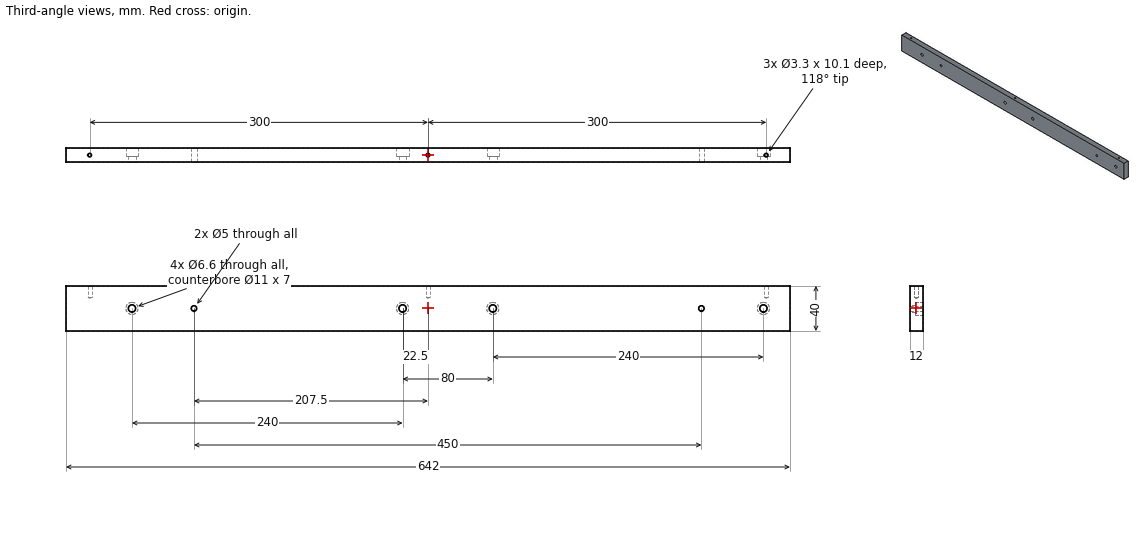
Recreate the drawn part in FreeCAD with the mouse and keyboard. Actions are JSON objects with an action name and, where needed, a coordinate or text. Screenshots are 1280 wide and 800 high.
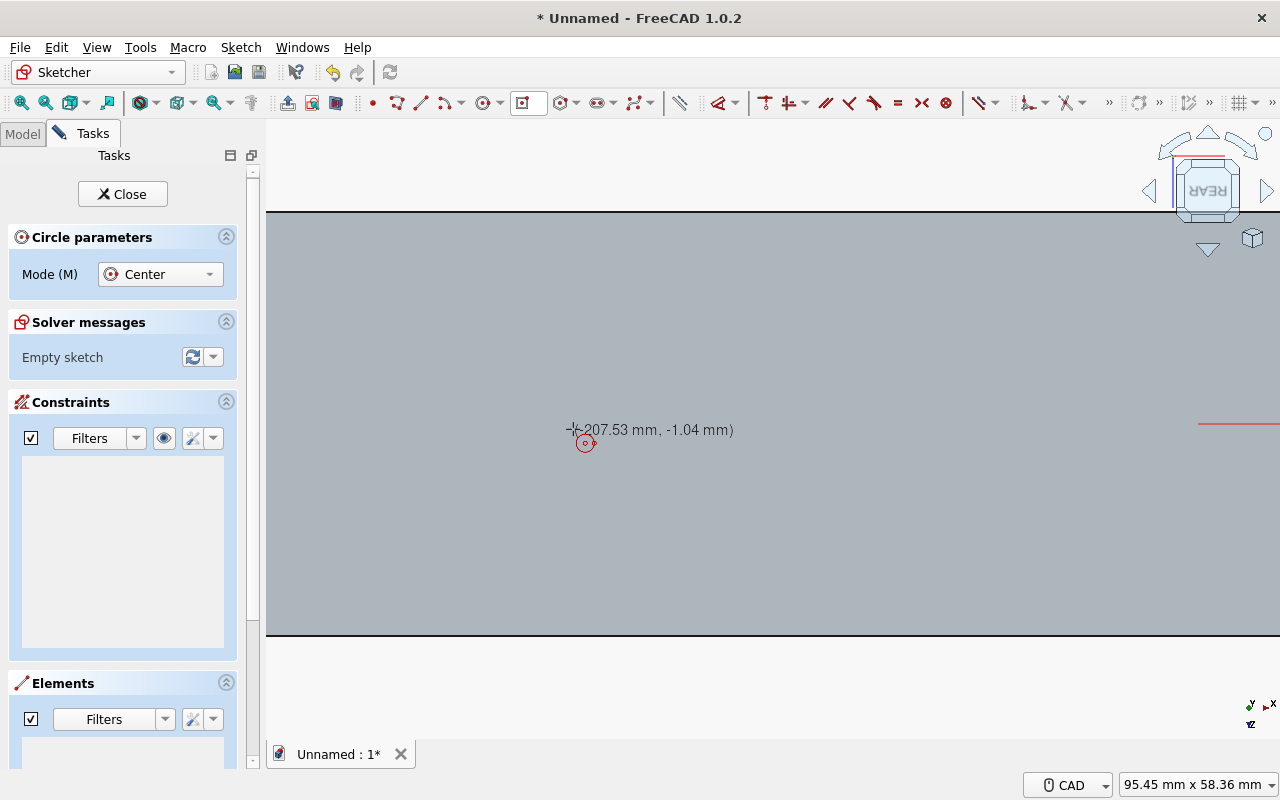
{"action": "scroll", "coordinate": [423, 430], "scroll_direction": "down", "scroll_amount": 11}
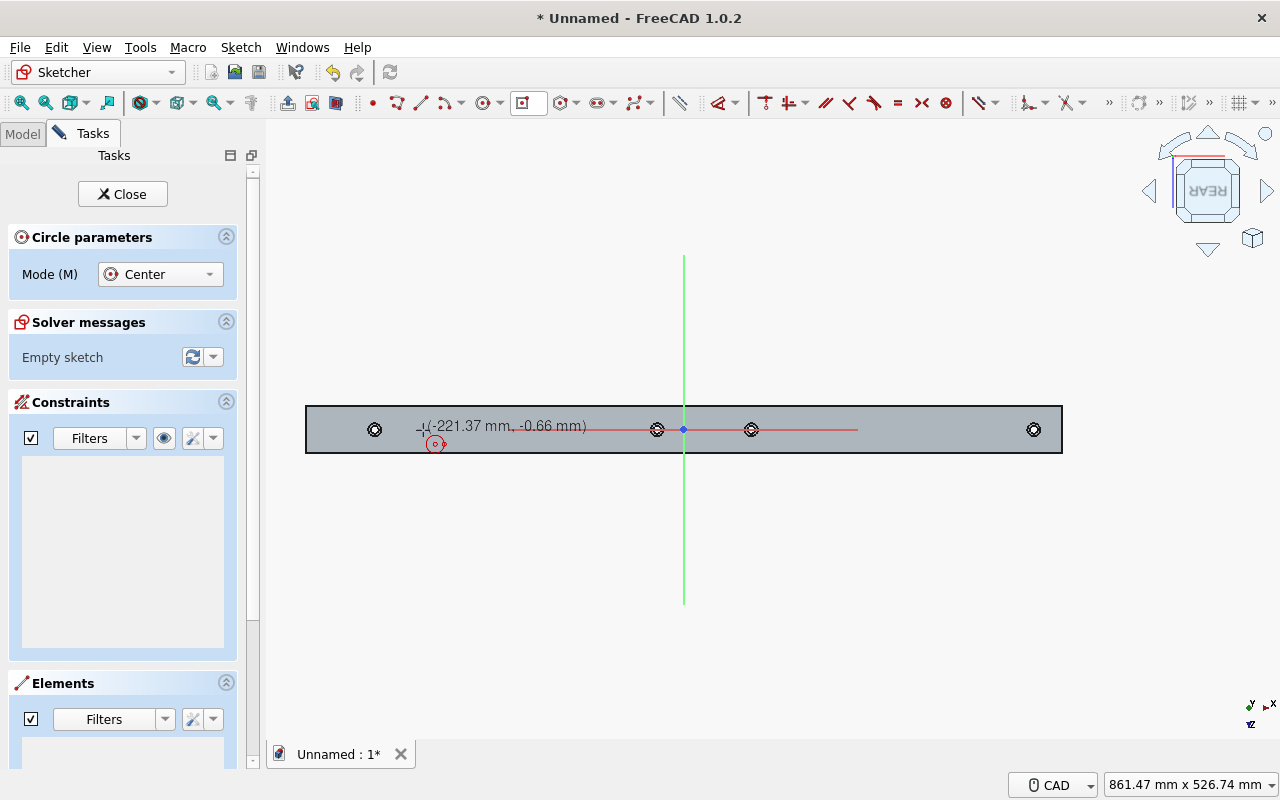
{"action": "left_click", "coordinate": [439, 430]}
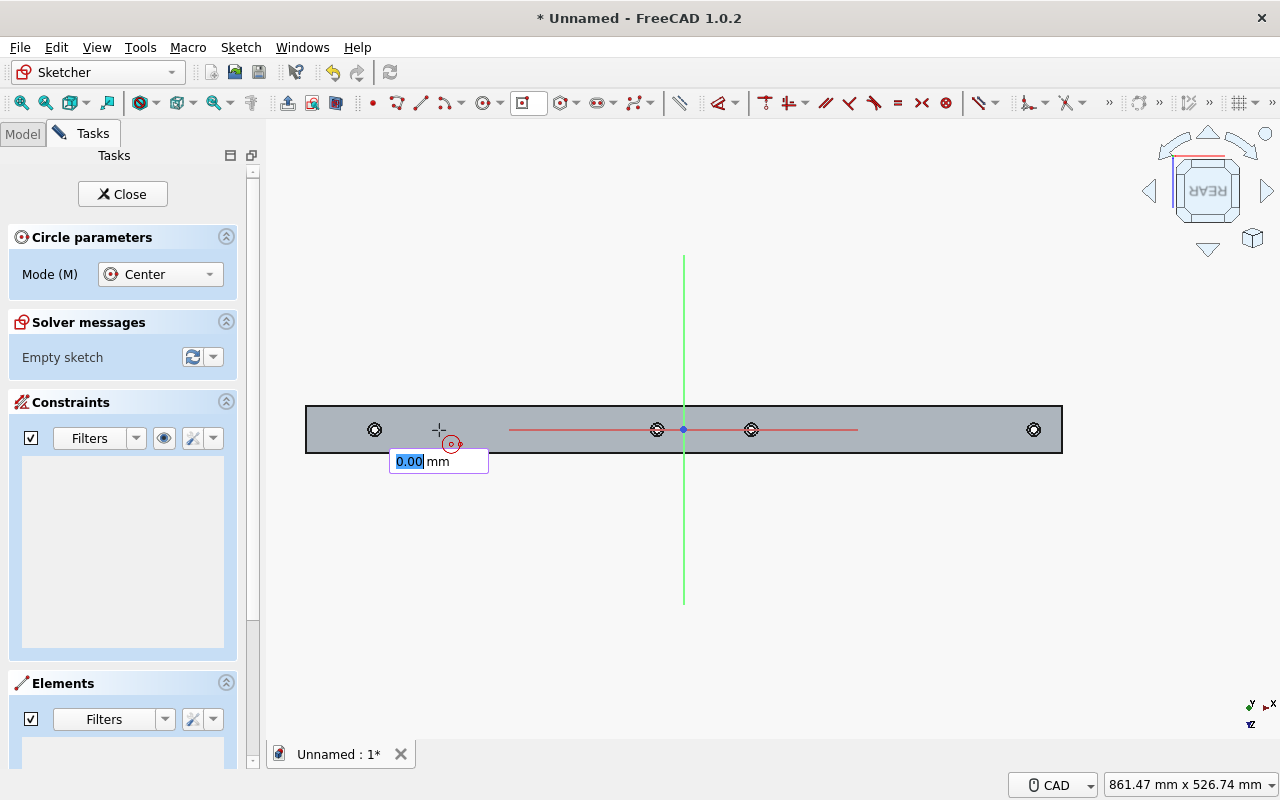
{"action": "scroll", "coordinate": [438, 433], "scroll_direction": "up", "scroll_amount": 9}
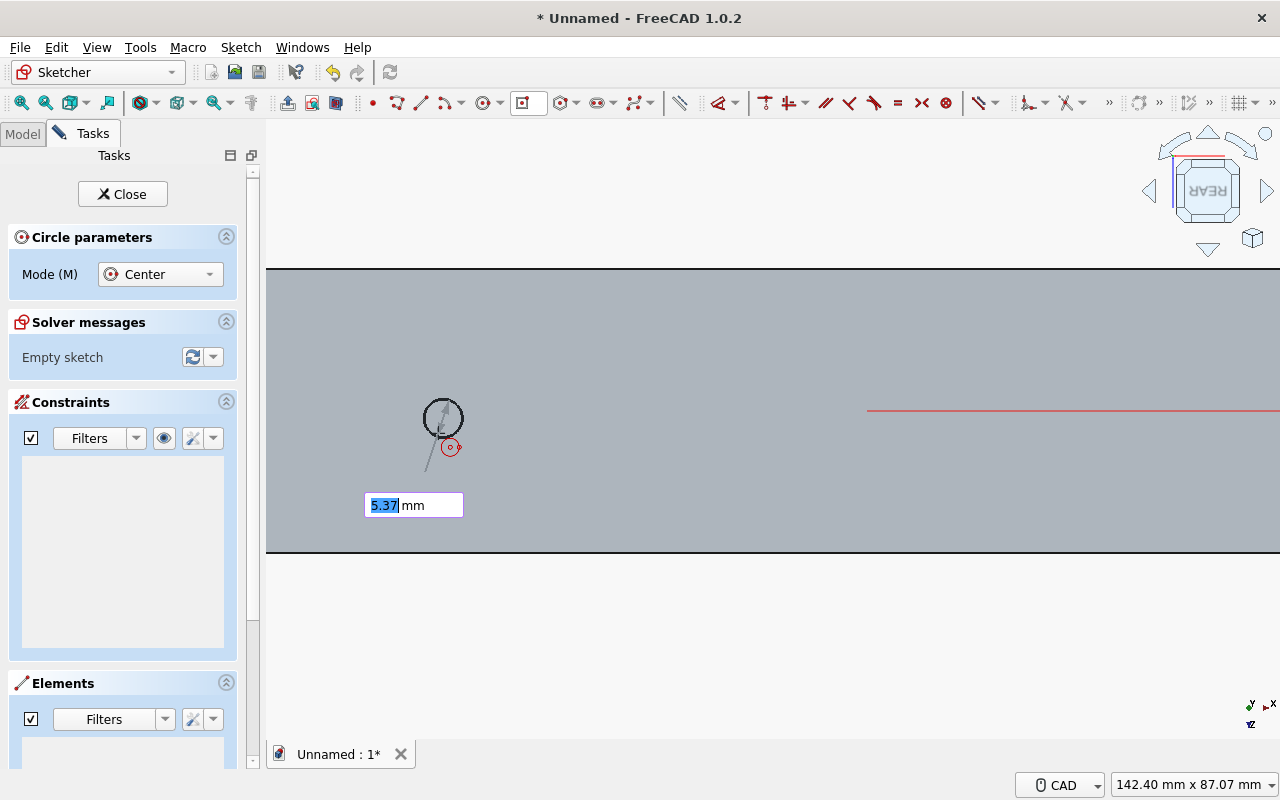
{"action": "left_click", "coordinate": [440, 428]}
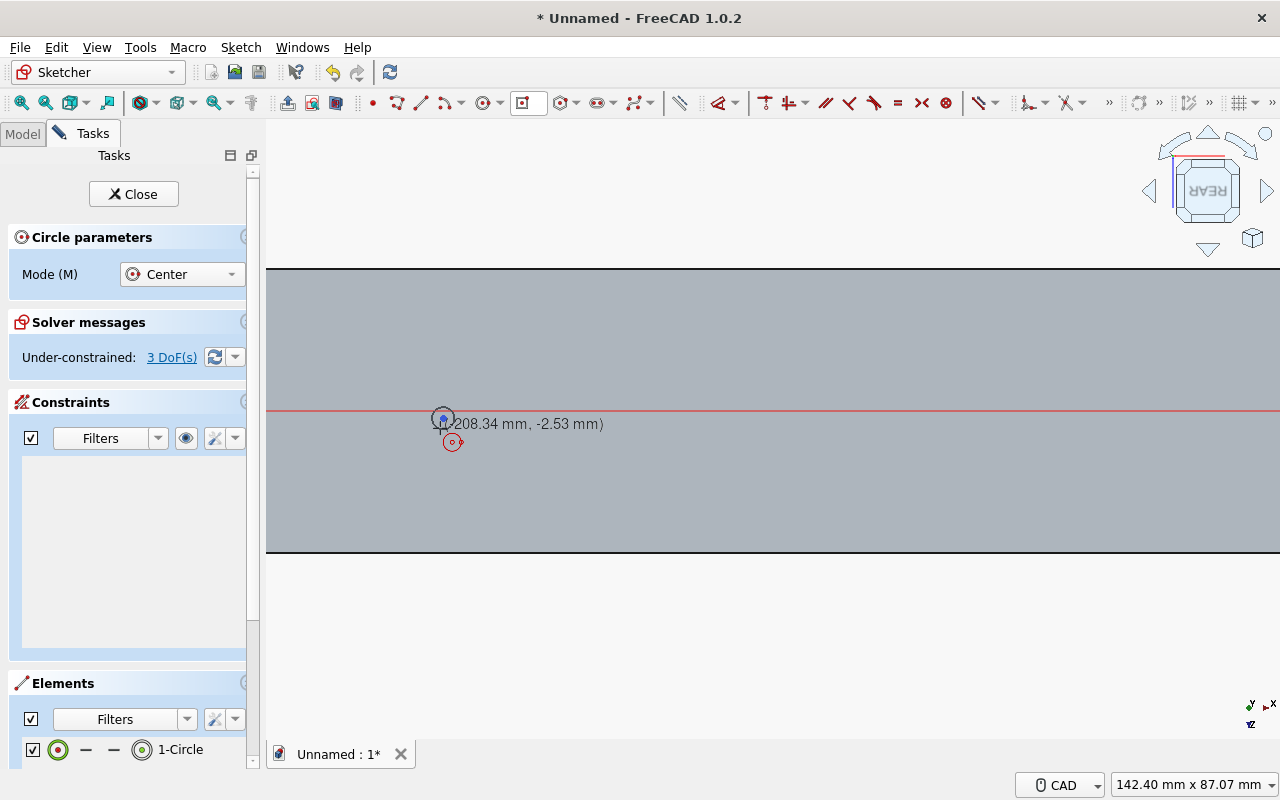
{"action": "scroll", "coordinate": [438, 433], "scroll_direction": "down", "scroll_amount": 9}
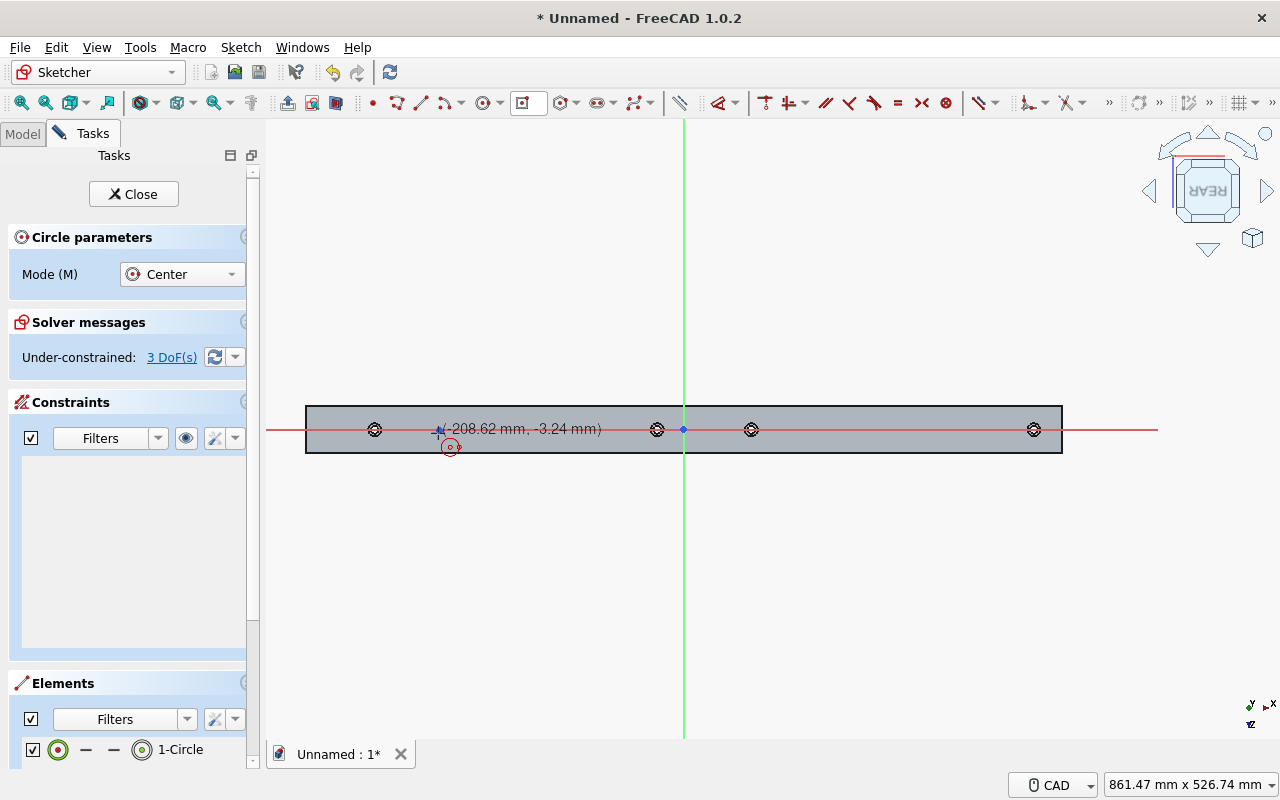
{"action": "scroll", "coordinate": [969, 430], "scroll_direction": "up", "scroll_amount": 11}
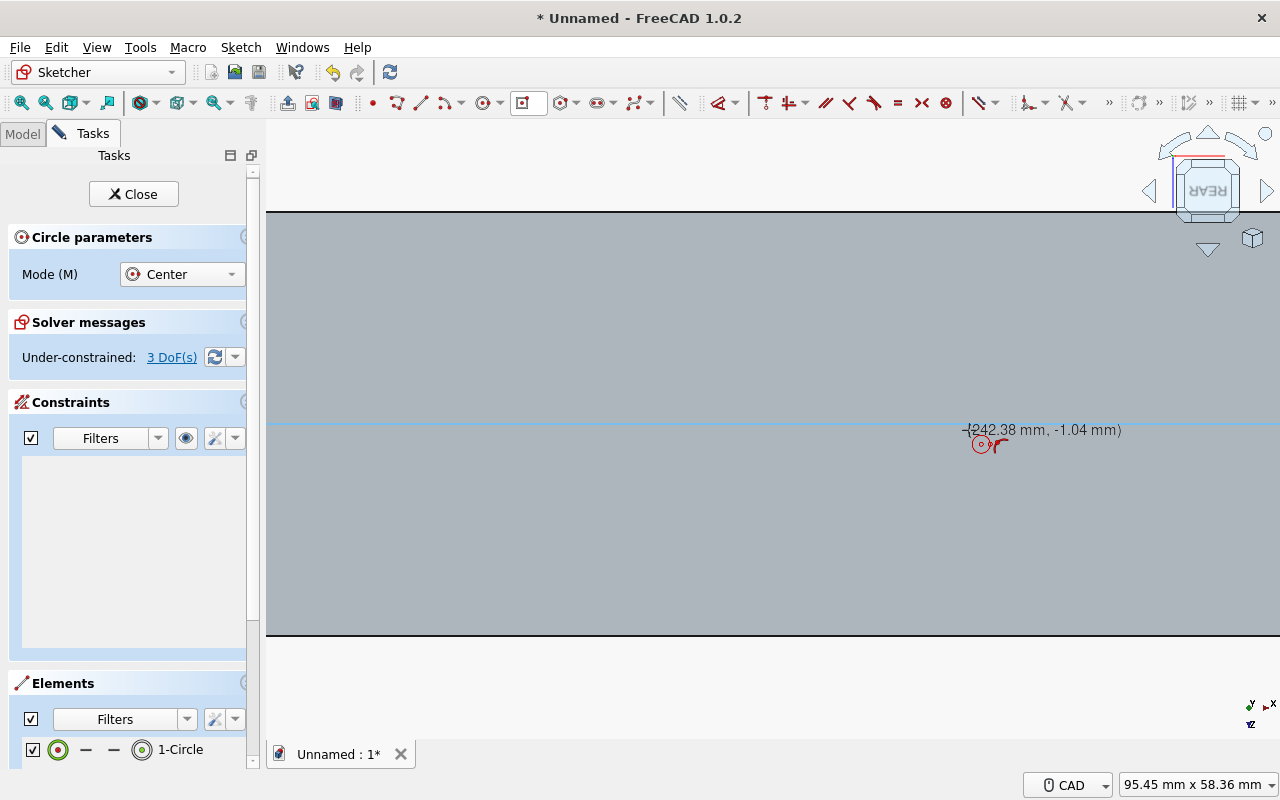
{"action": "scroll", "coordinate": [970, 430], "scroll_direction": "down", "scroll_amount": 11}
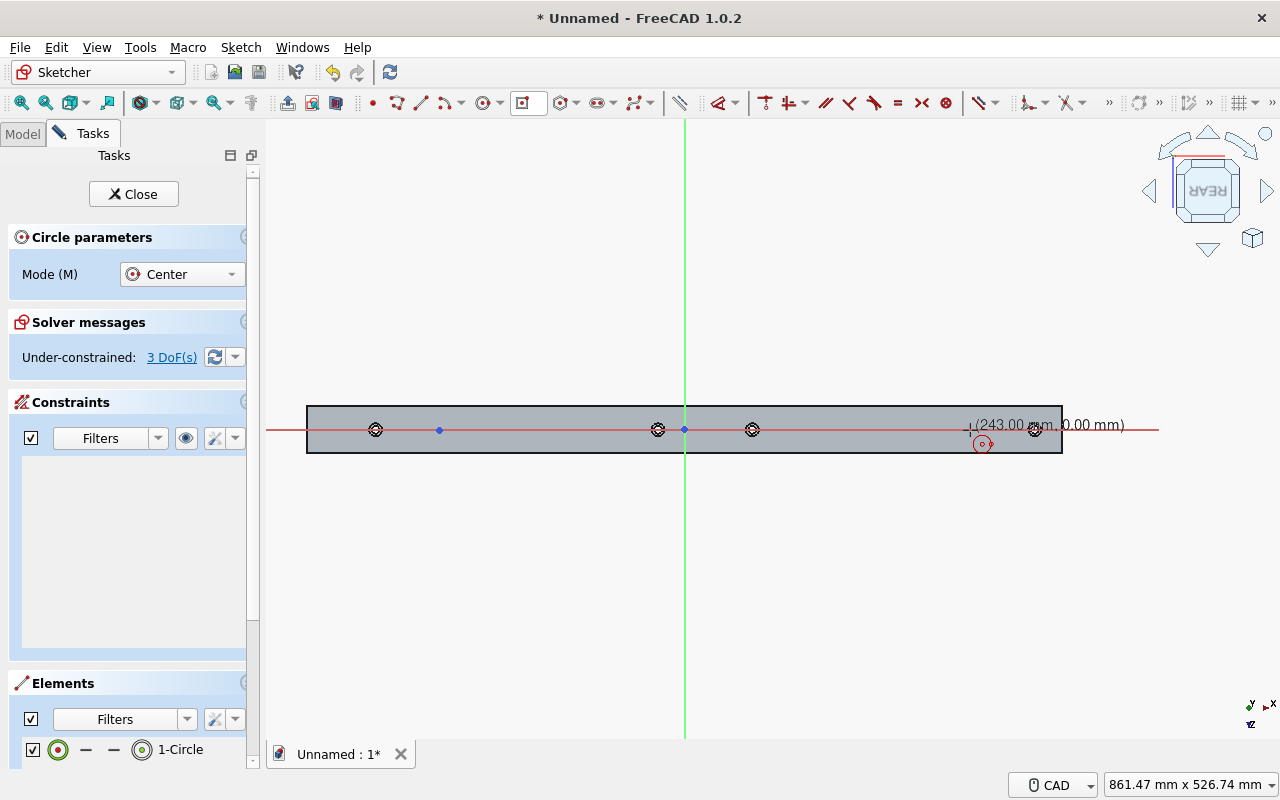
{"action": "left_click", "coordinate": [970, 430]}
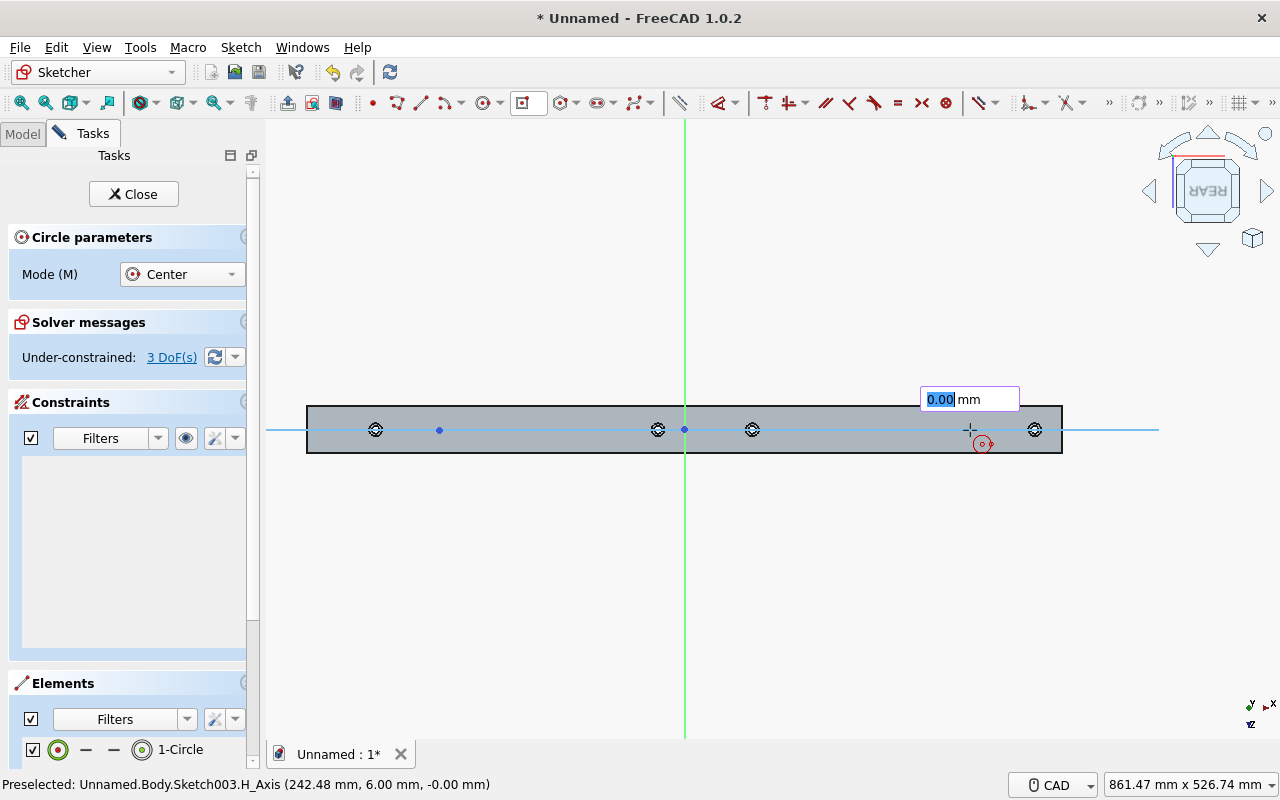
{"action": "scroll", "coordinate": [969, 433], "scroll_direction": "up", "scroll_amount": 9}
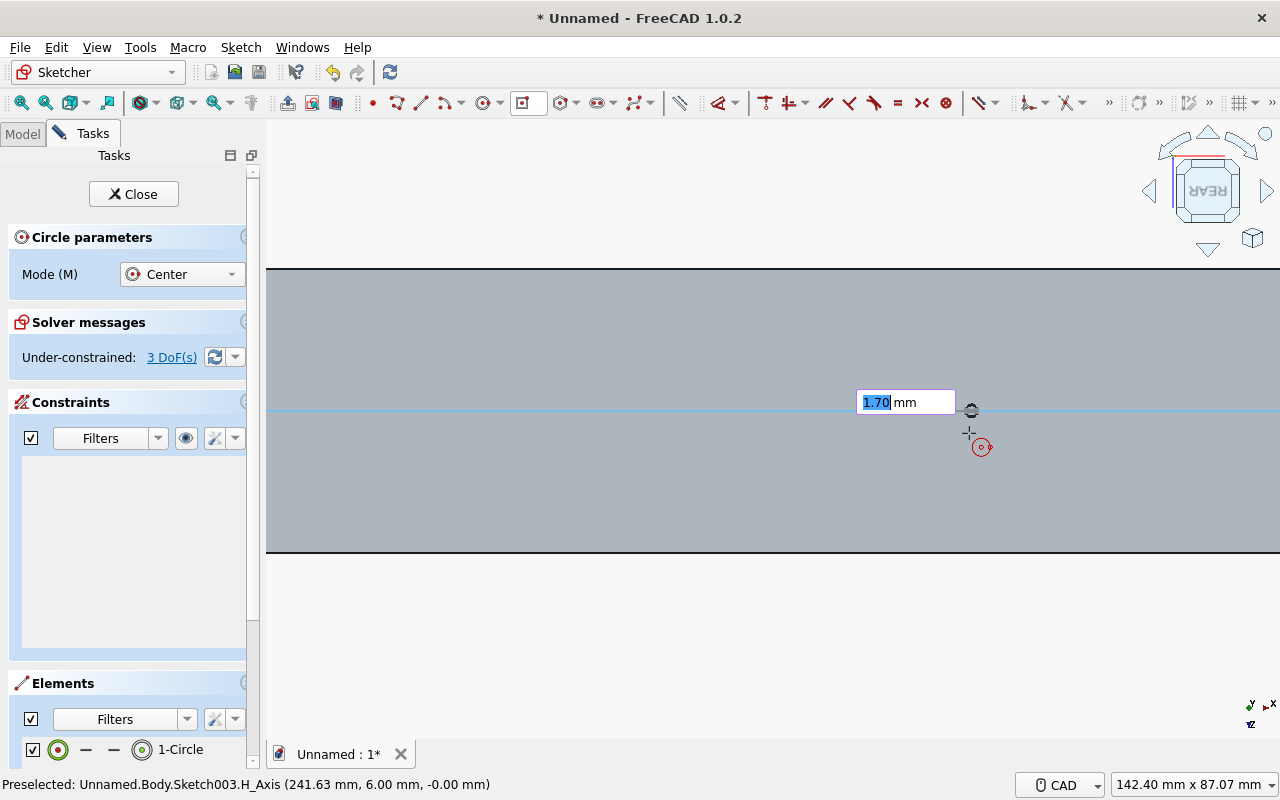
{"action": "left_click", "coordinate": [966, 428]}
{"action": "key", "text": "Escape"}